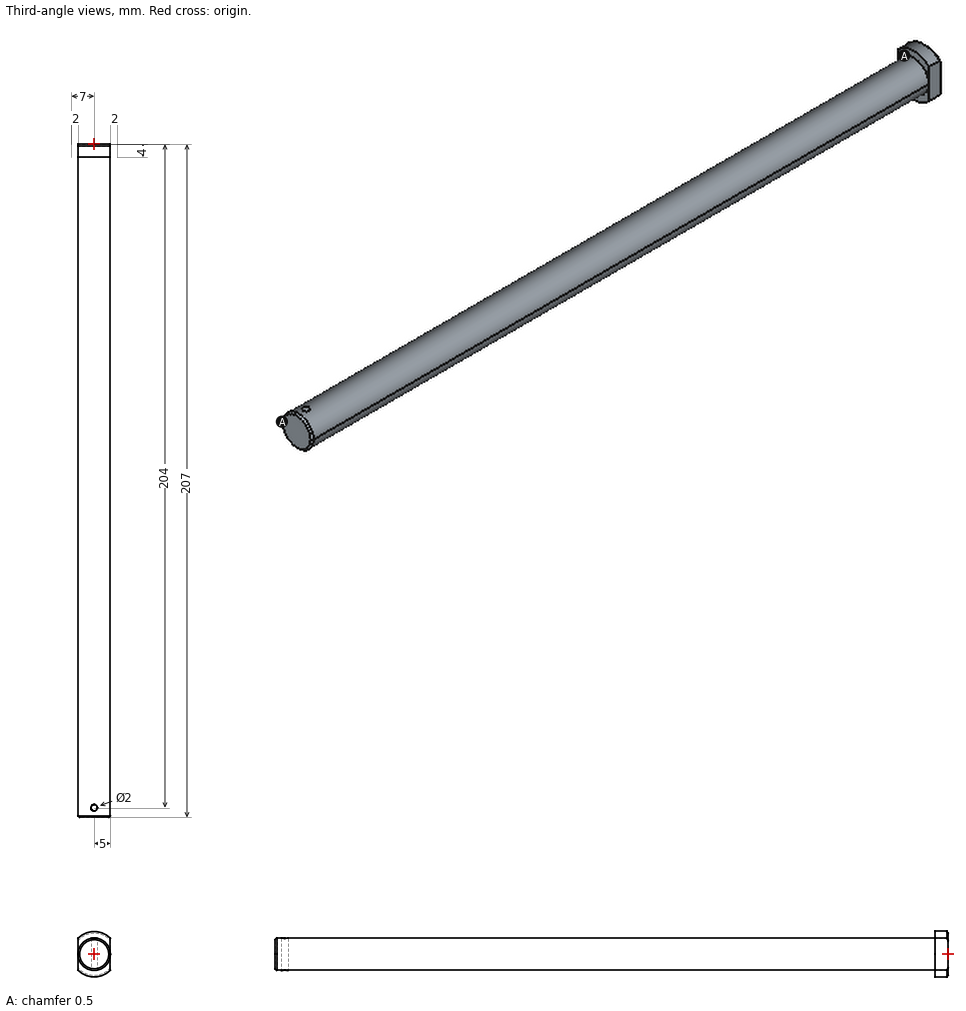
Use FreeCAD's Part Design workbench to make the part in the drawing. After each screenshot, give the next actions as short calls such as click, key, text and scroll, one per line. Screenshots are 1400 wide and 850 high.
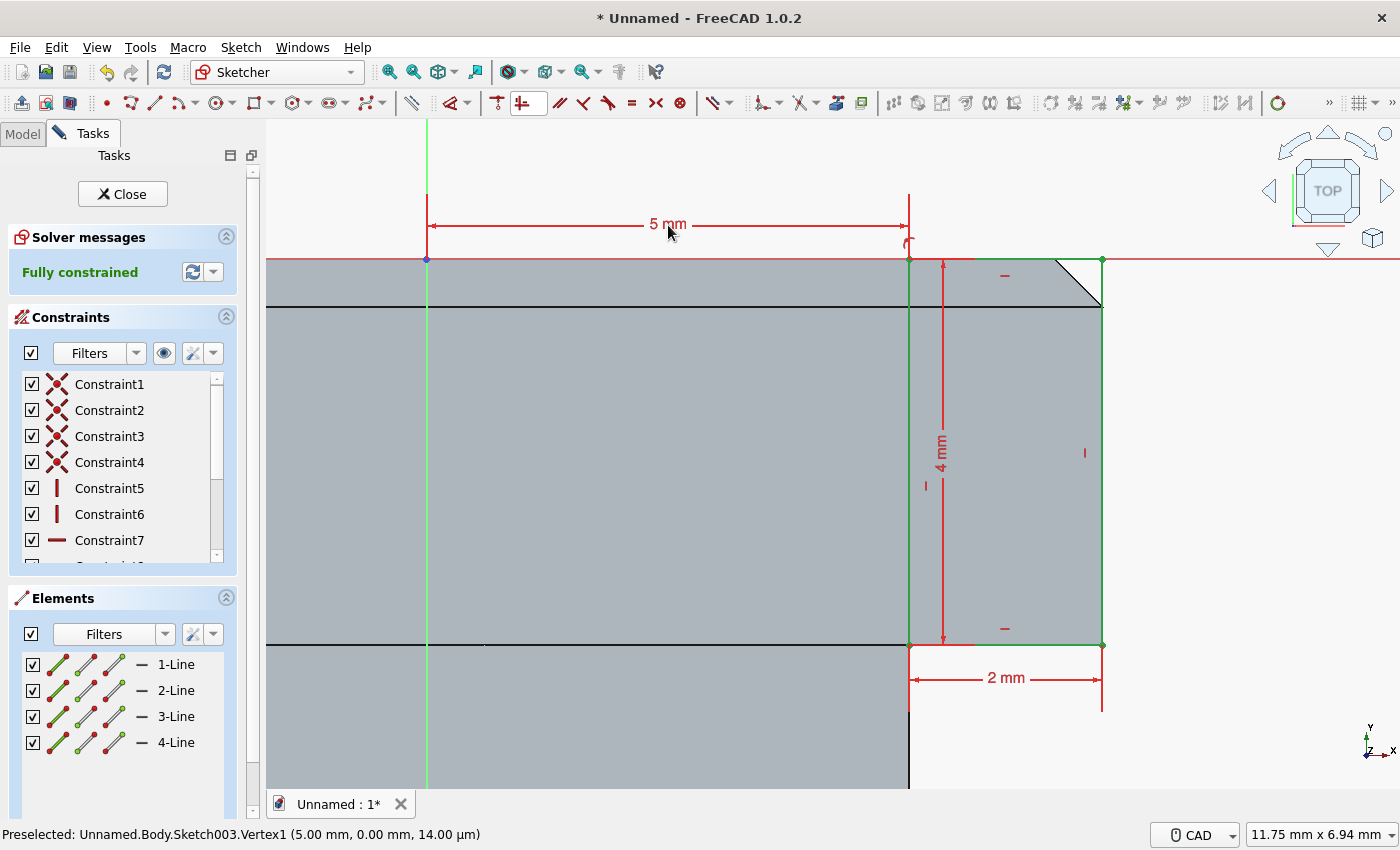
click(123, 194)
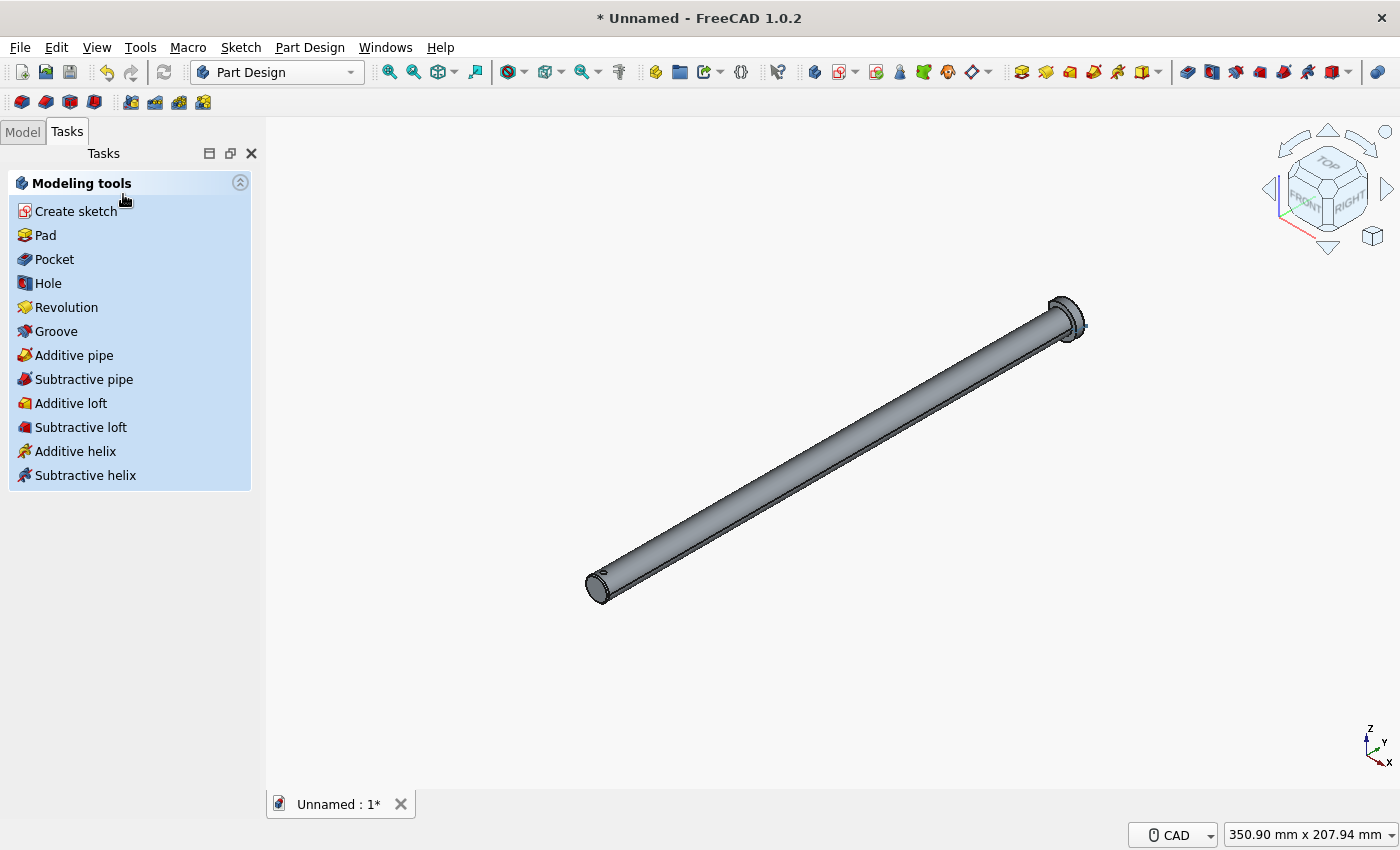
click(1188, 72)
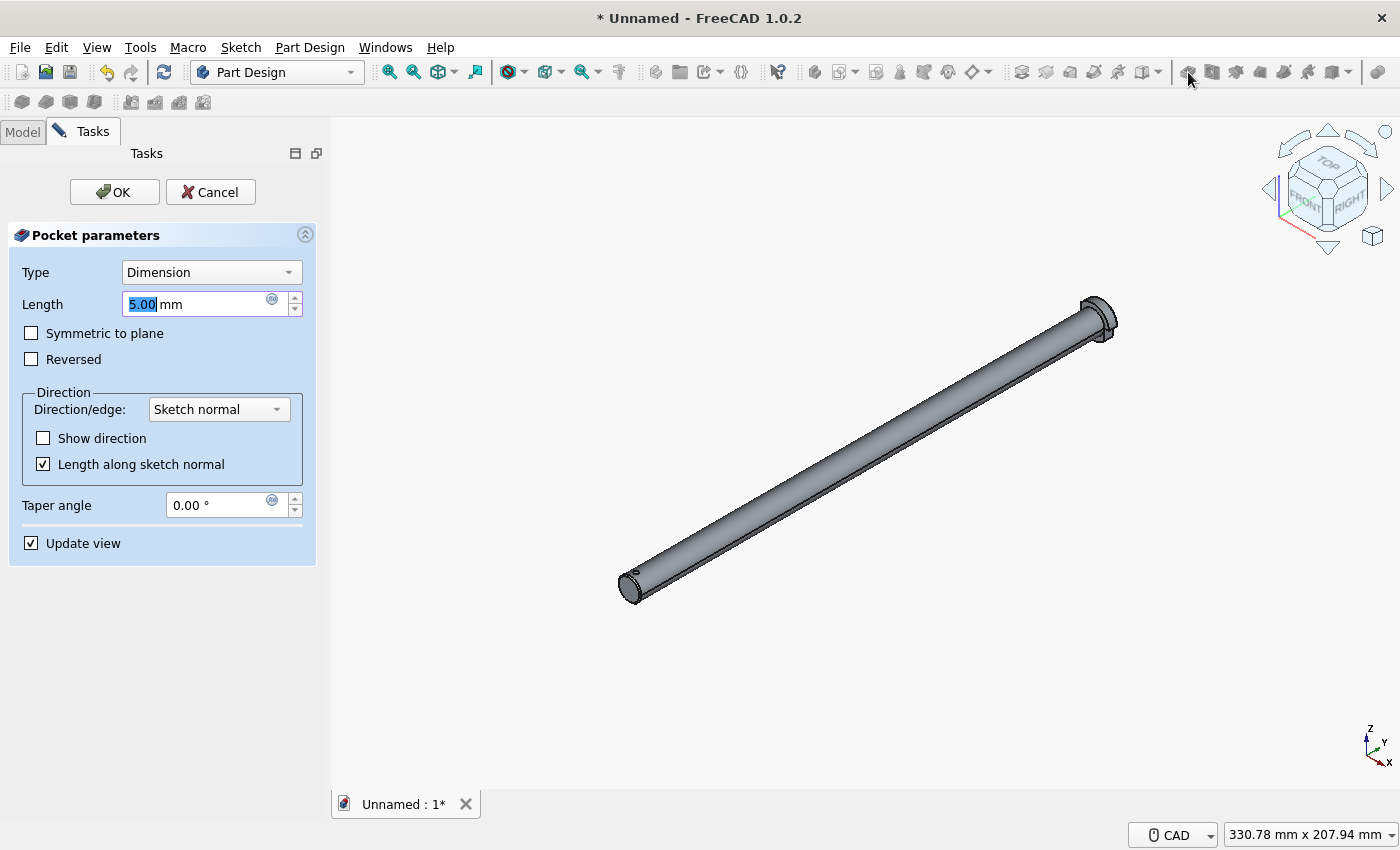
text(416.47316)
key(Tab)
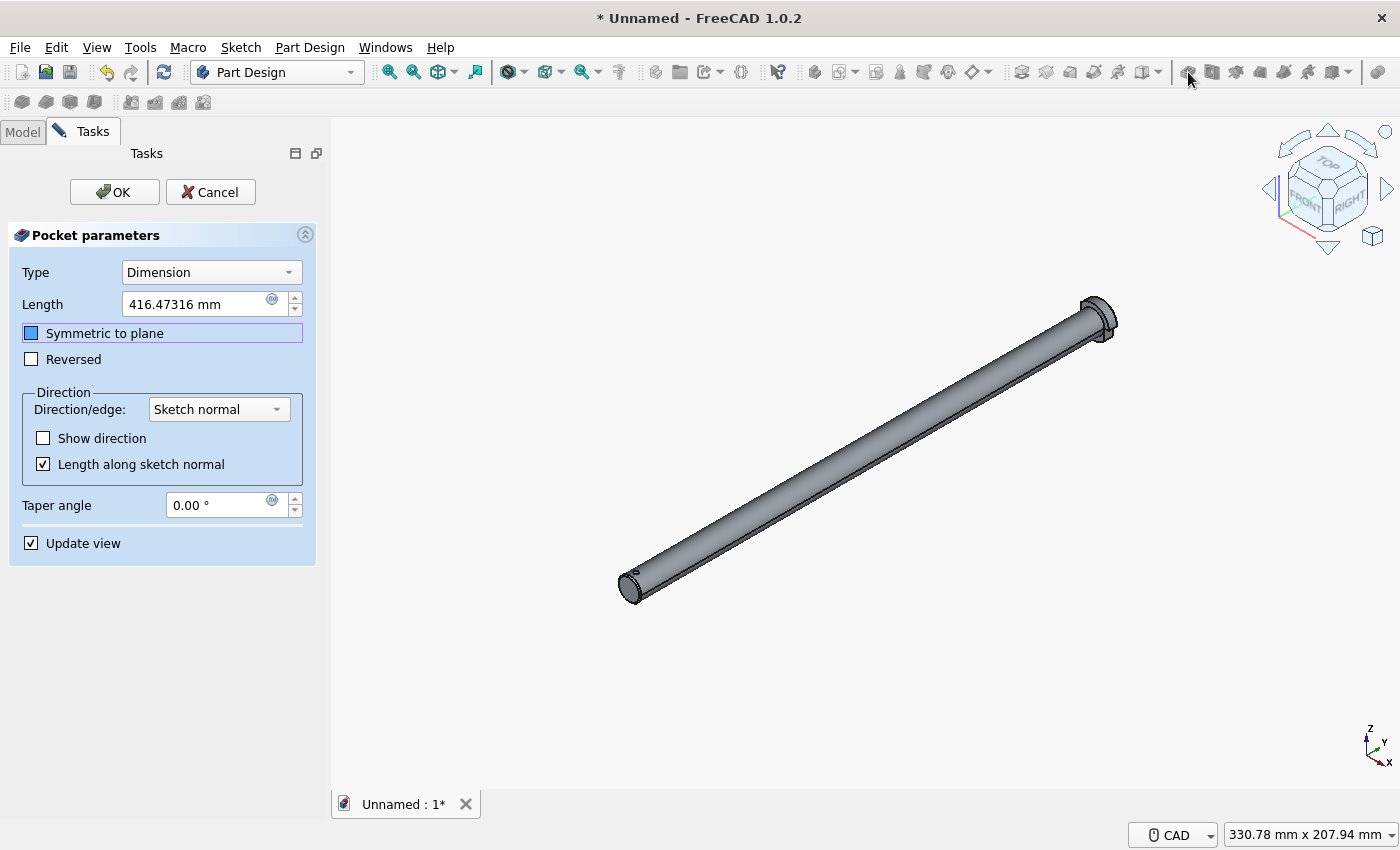
click(30, 333)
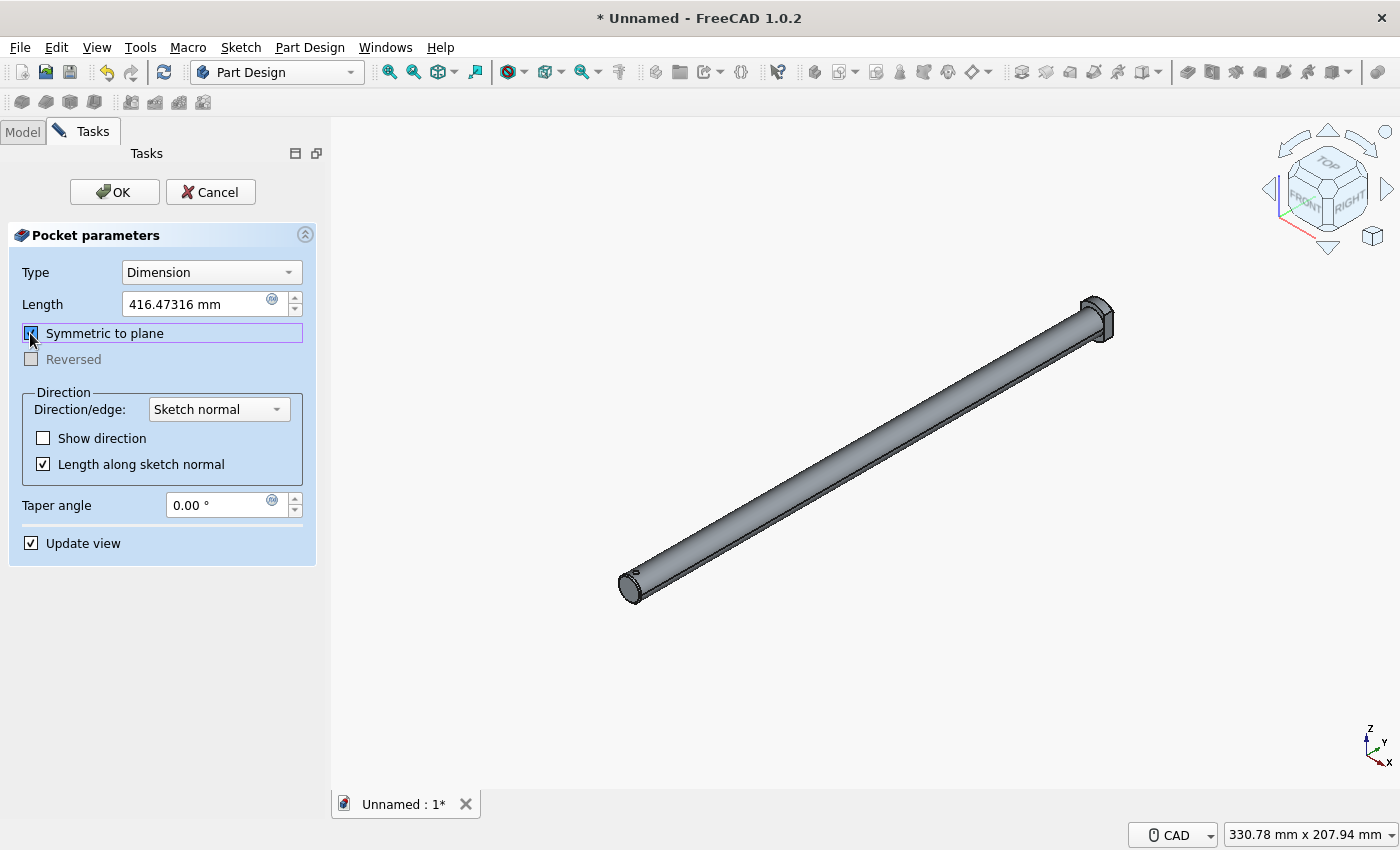
click(115, 192)